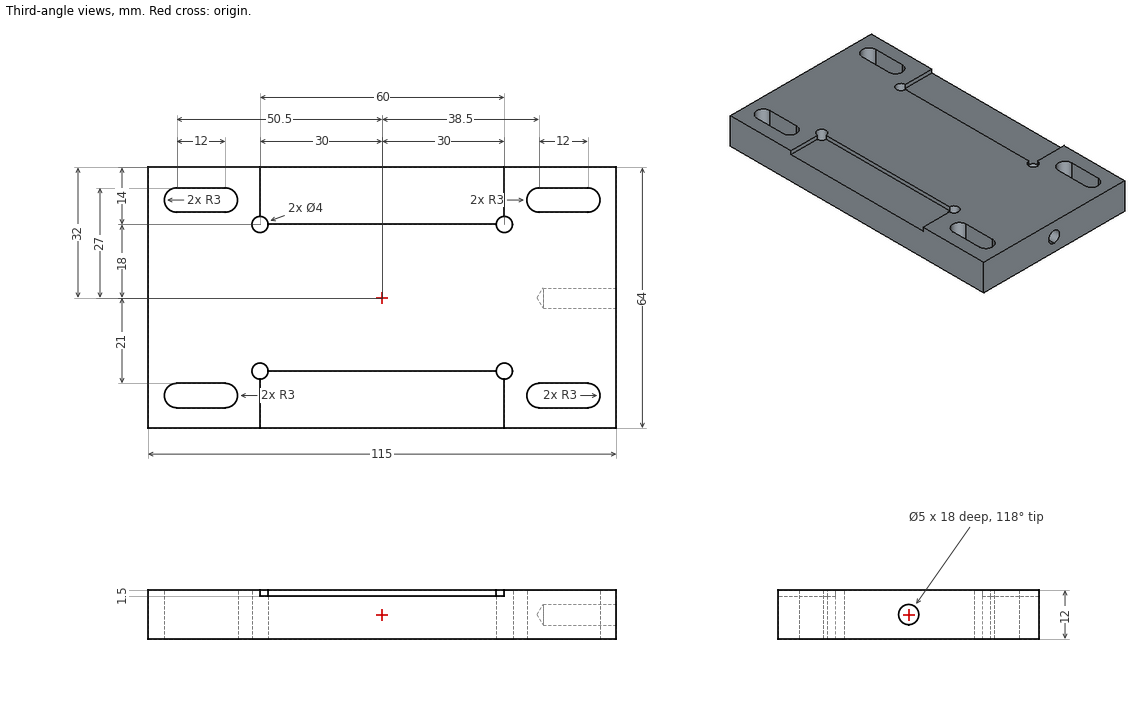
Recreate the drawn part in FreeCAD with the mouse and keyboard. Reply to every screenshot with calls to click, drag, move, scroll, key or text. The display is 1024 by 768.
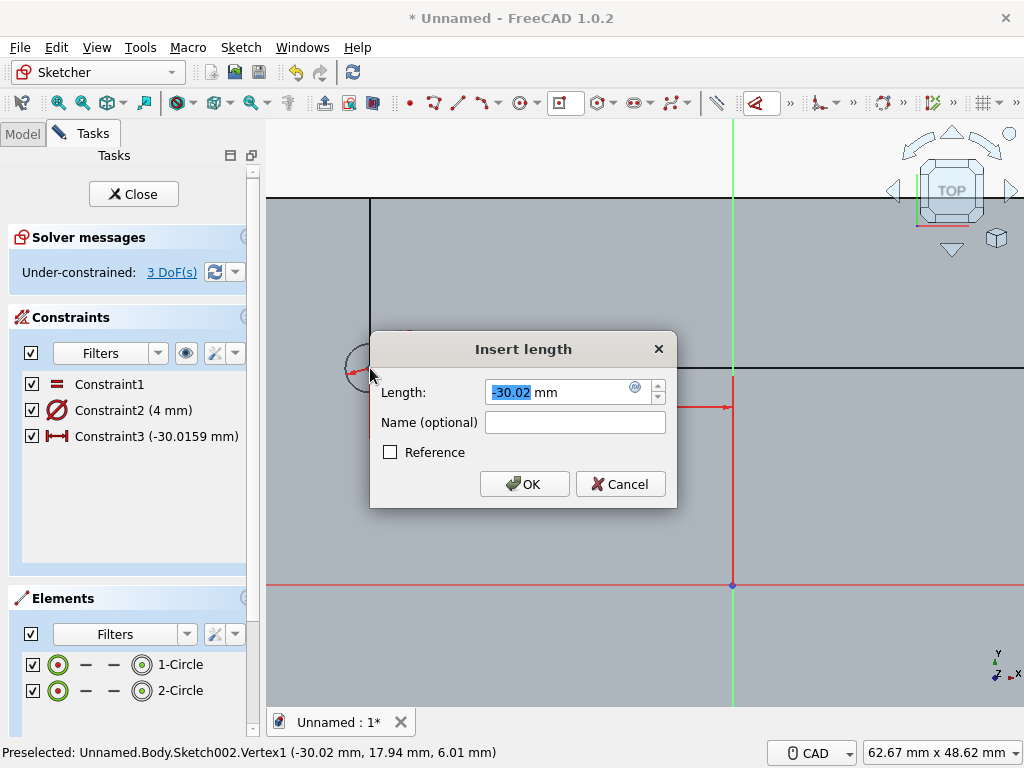
text(-30)
key(Return)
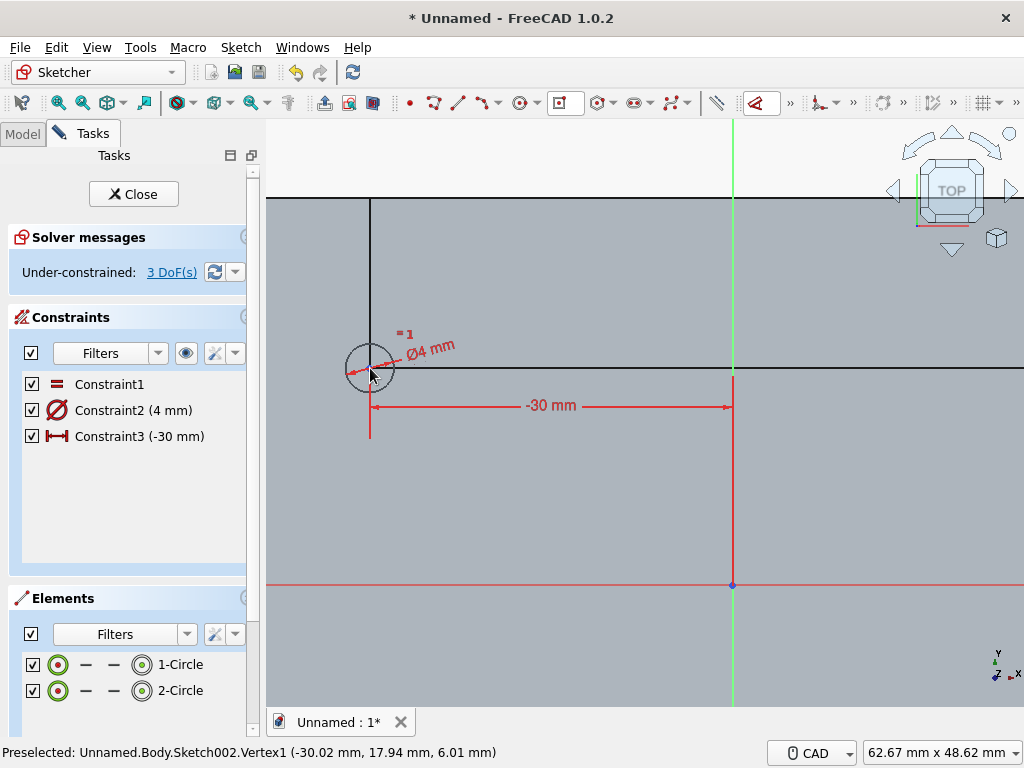
click(370, 368)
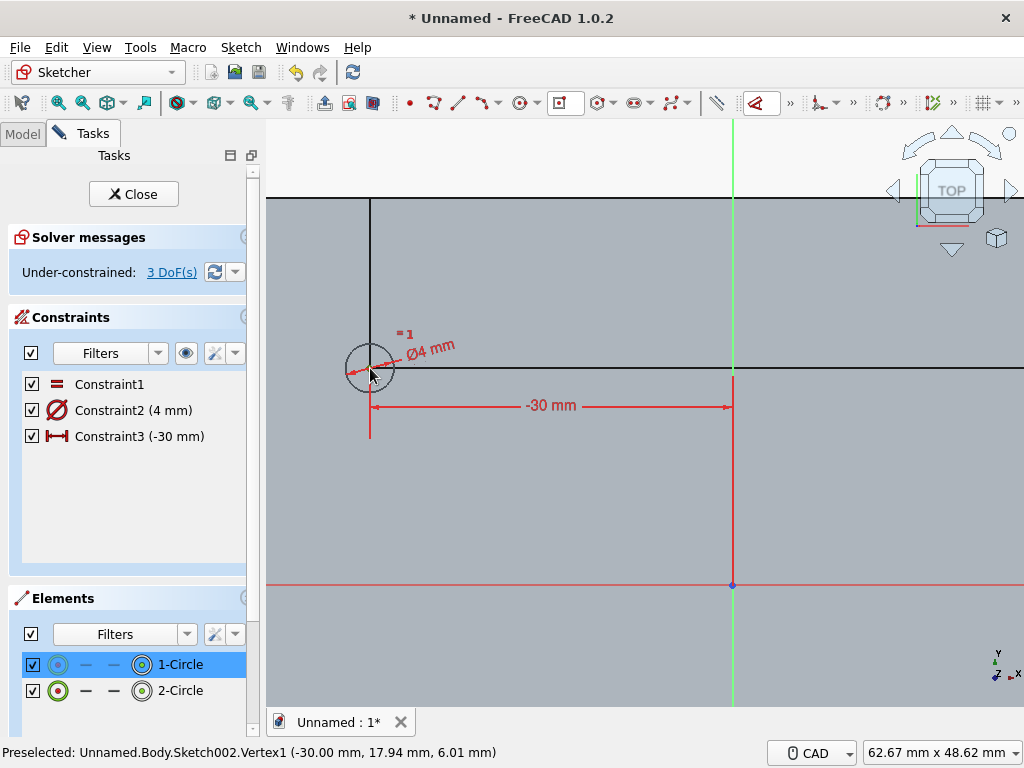
click(774, 104)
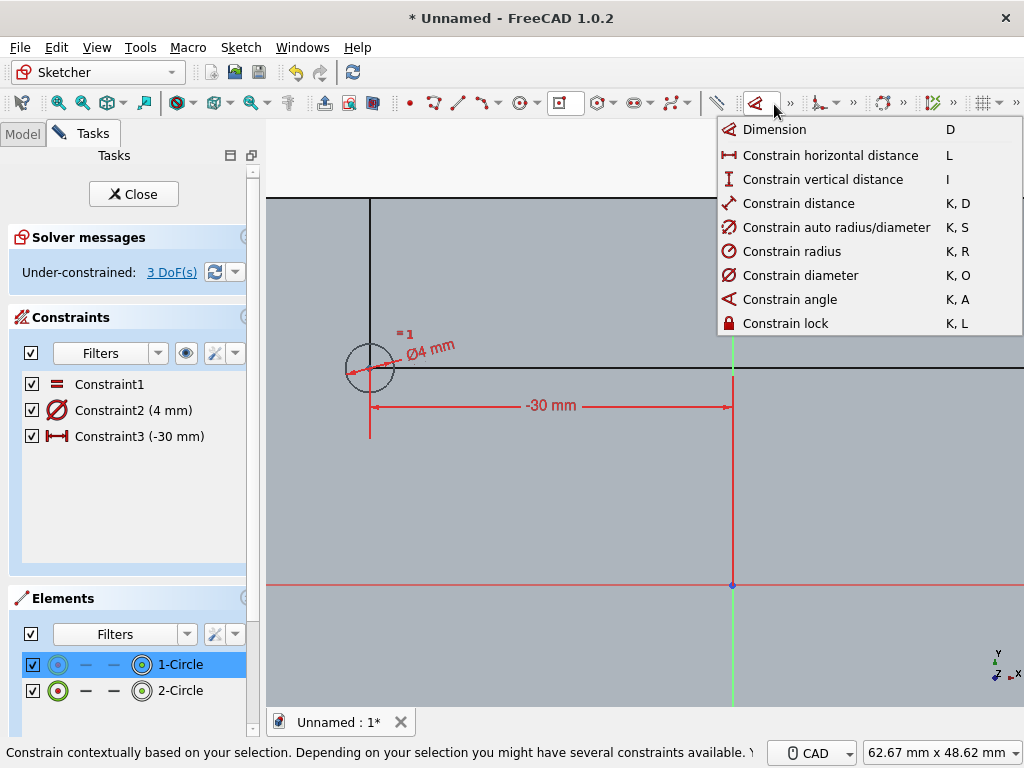
click(870, 179)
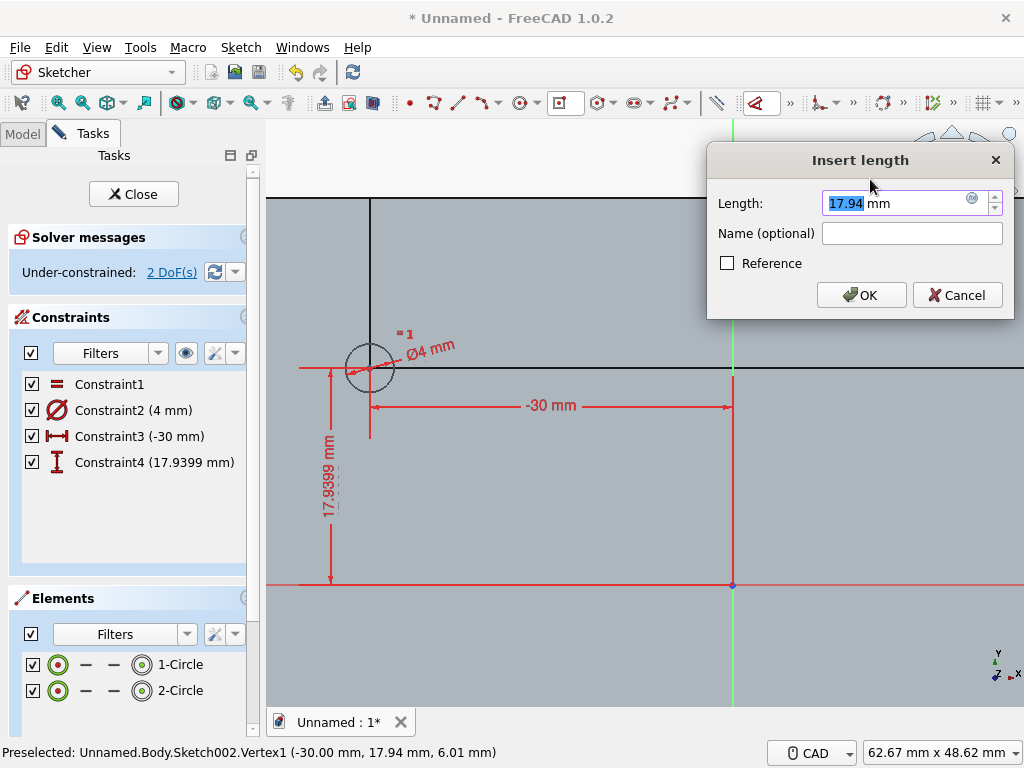
text(18)
key(Return)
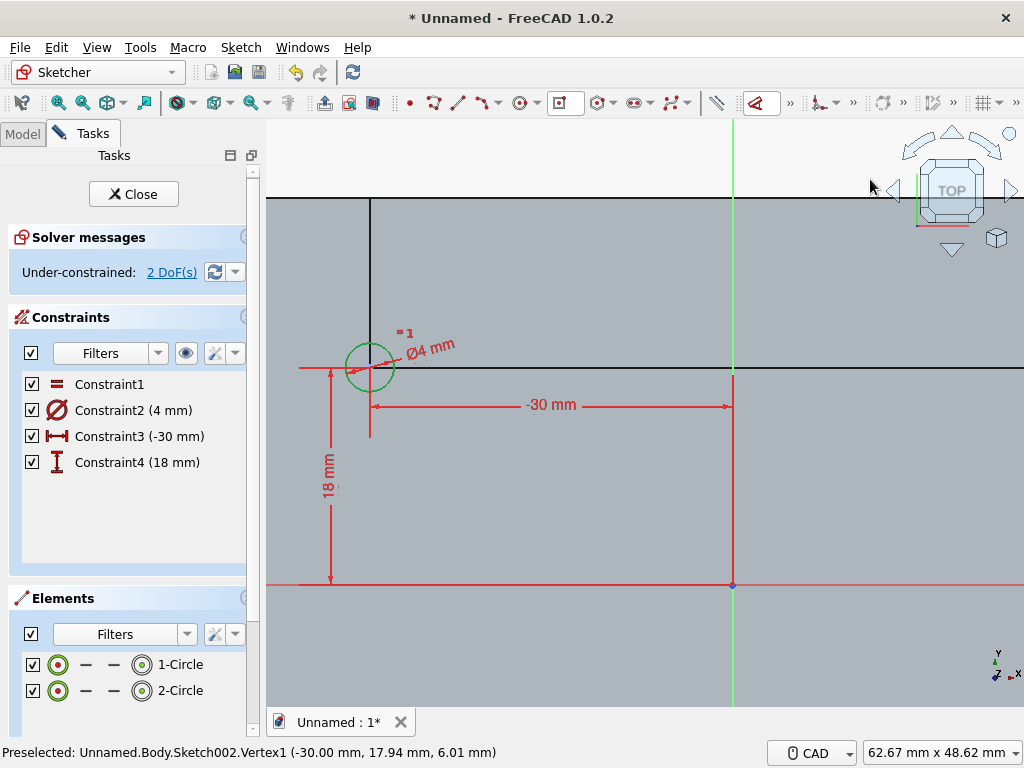
scroll(387, 351, down, 3)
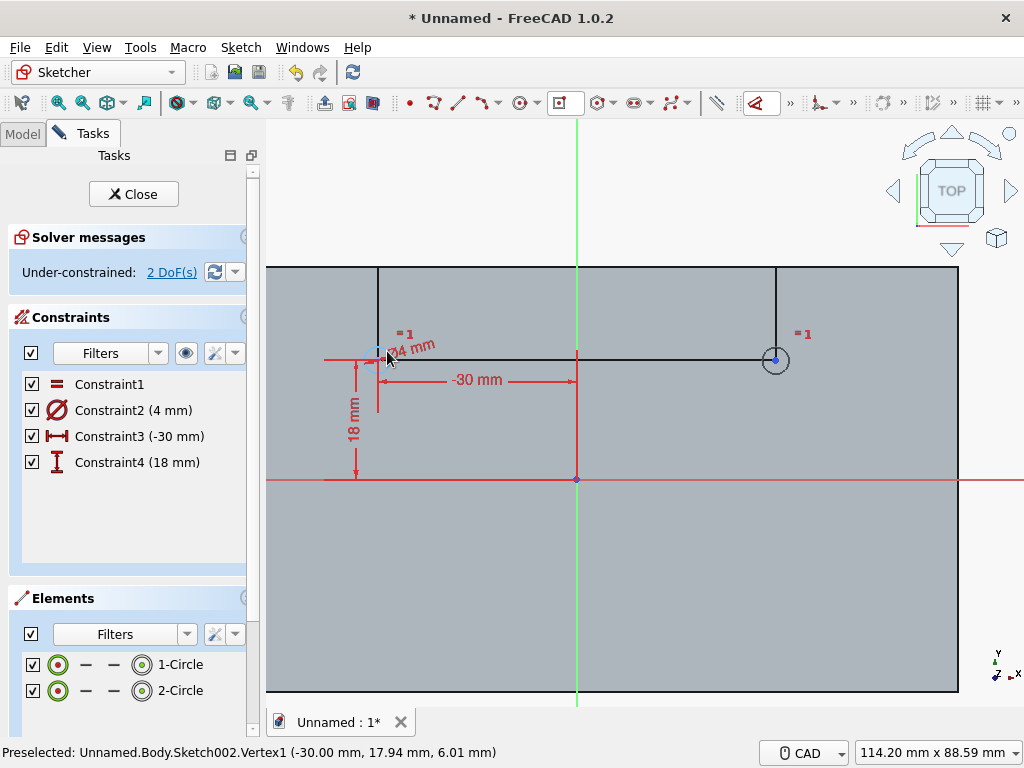
click(776, 361)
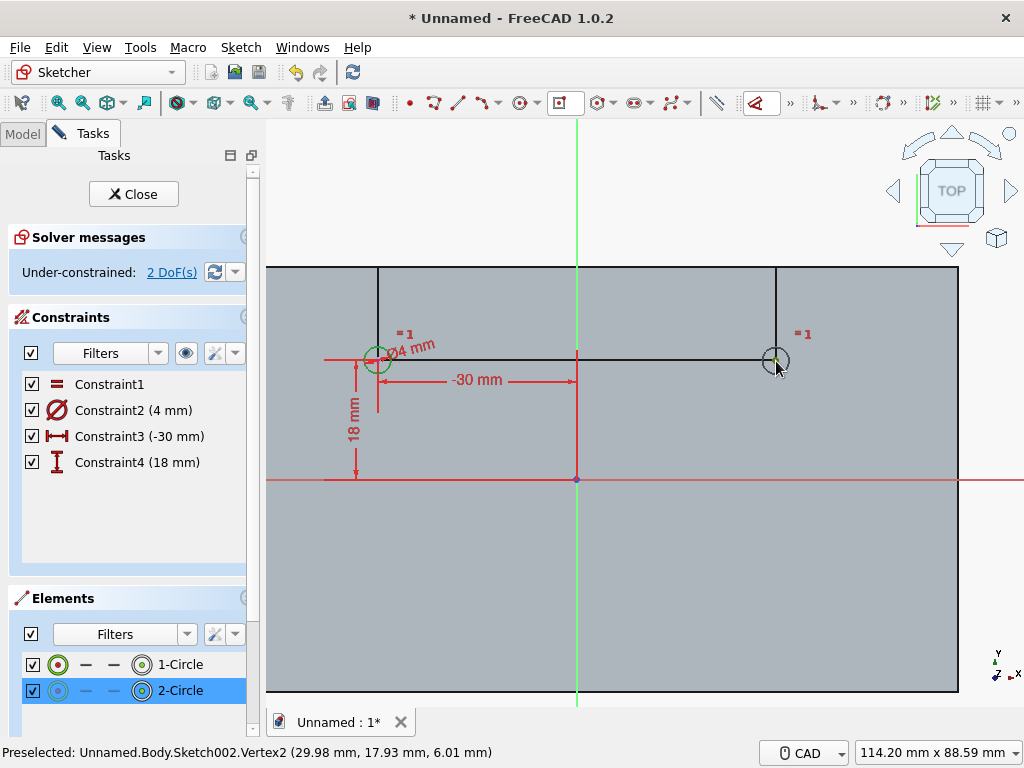
click(774, 104)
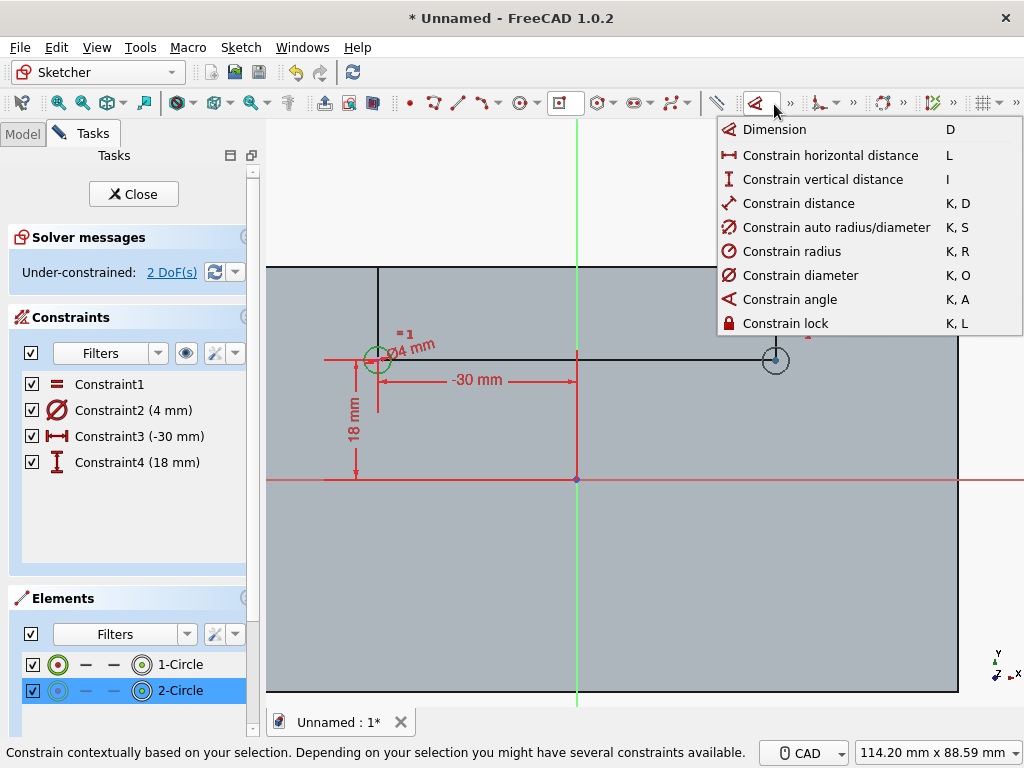
click(870, 155)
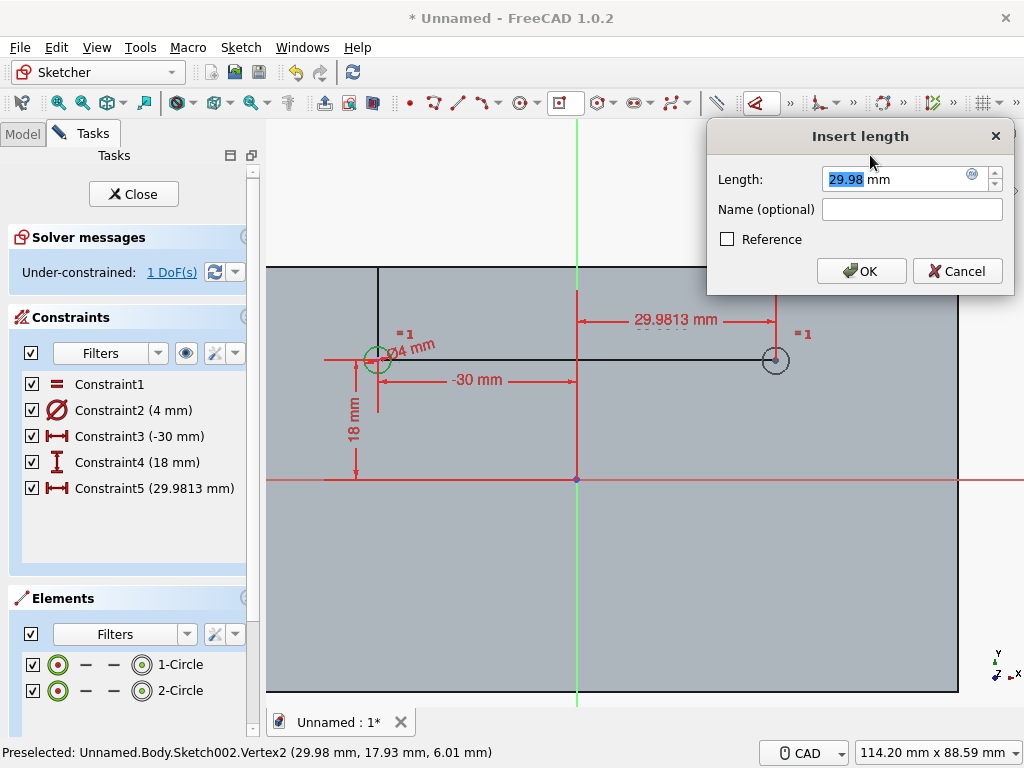
text(30)
key(Return)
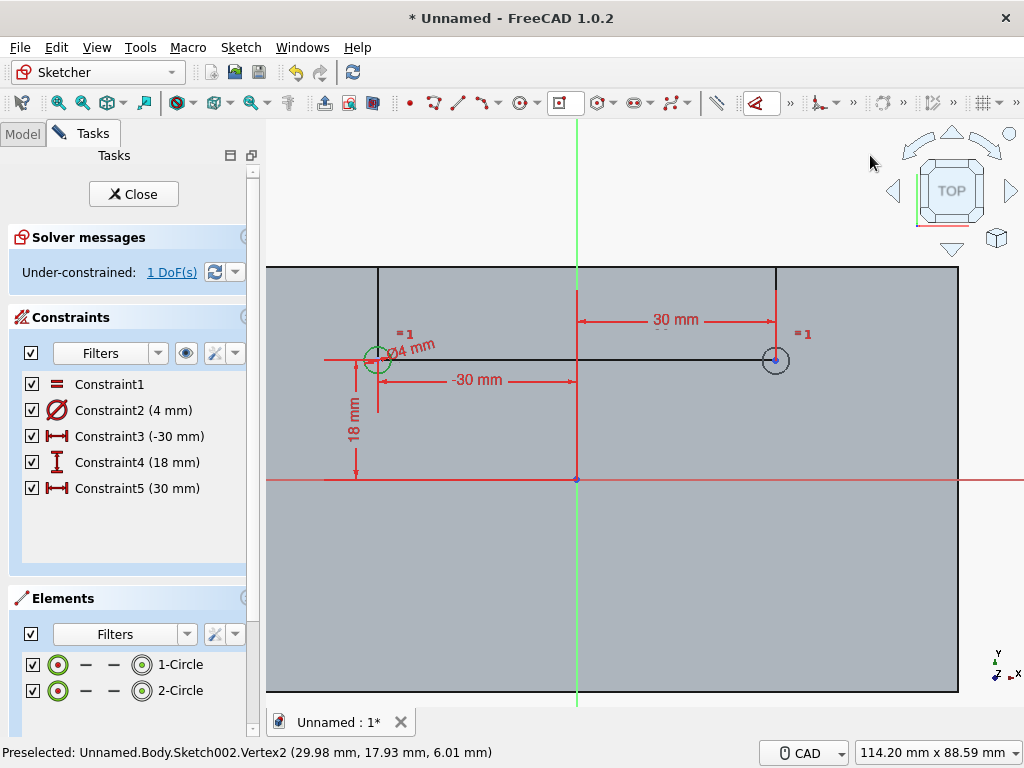
click(776, 361)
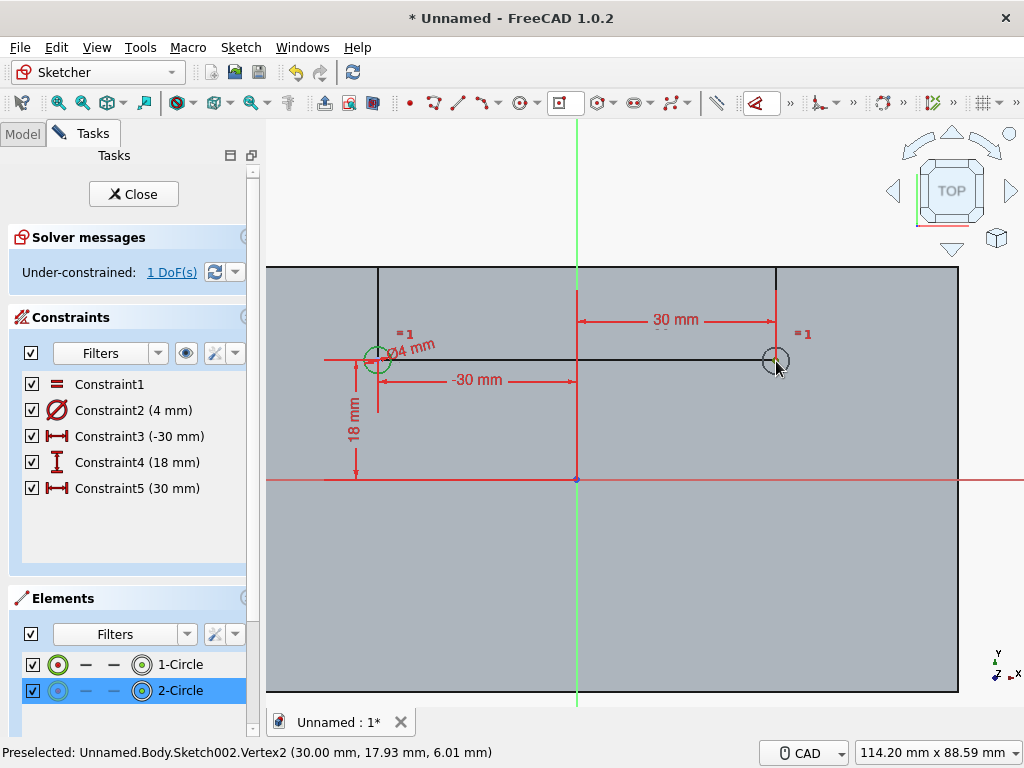
click(774, 104)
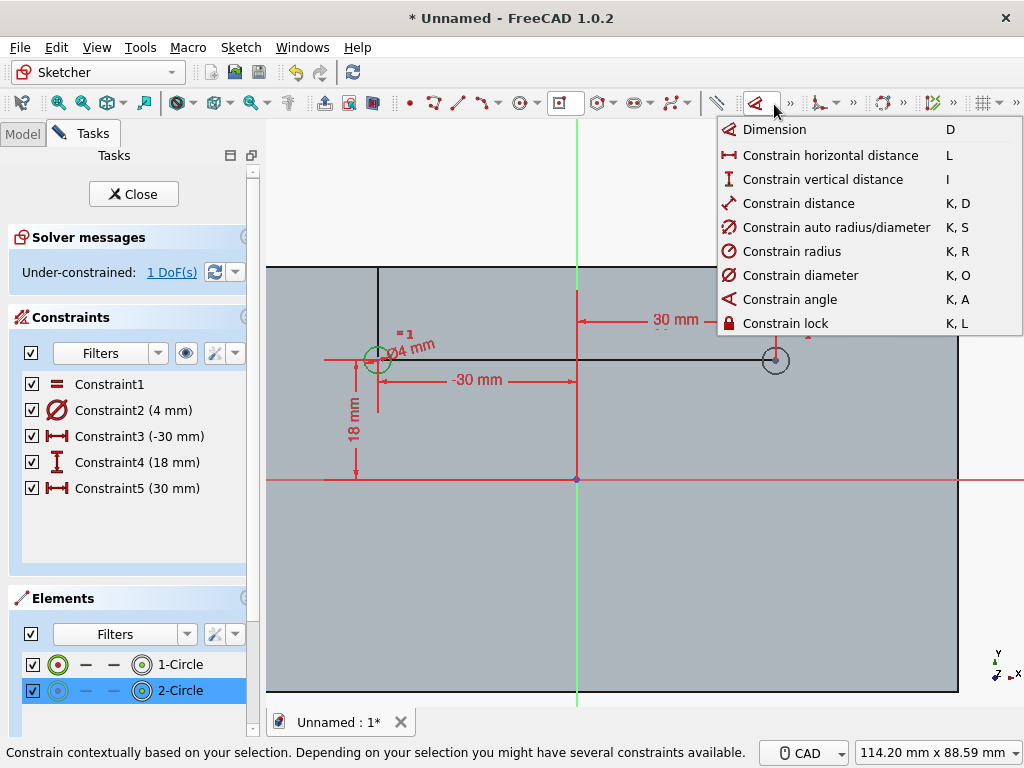
click(870, 179)